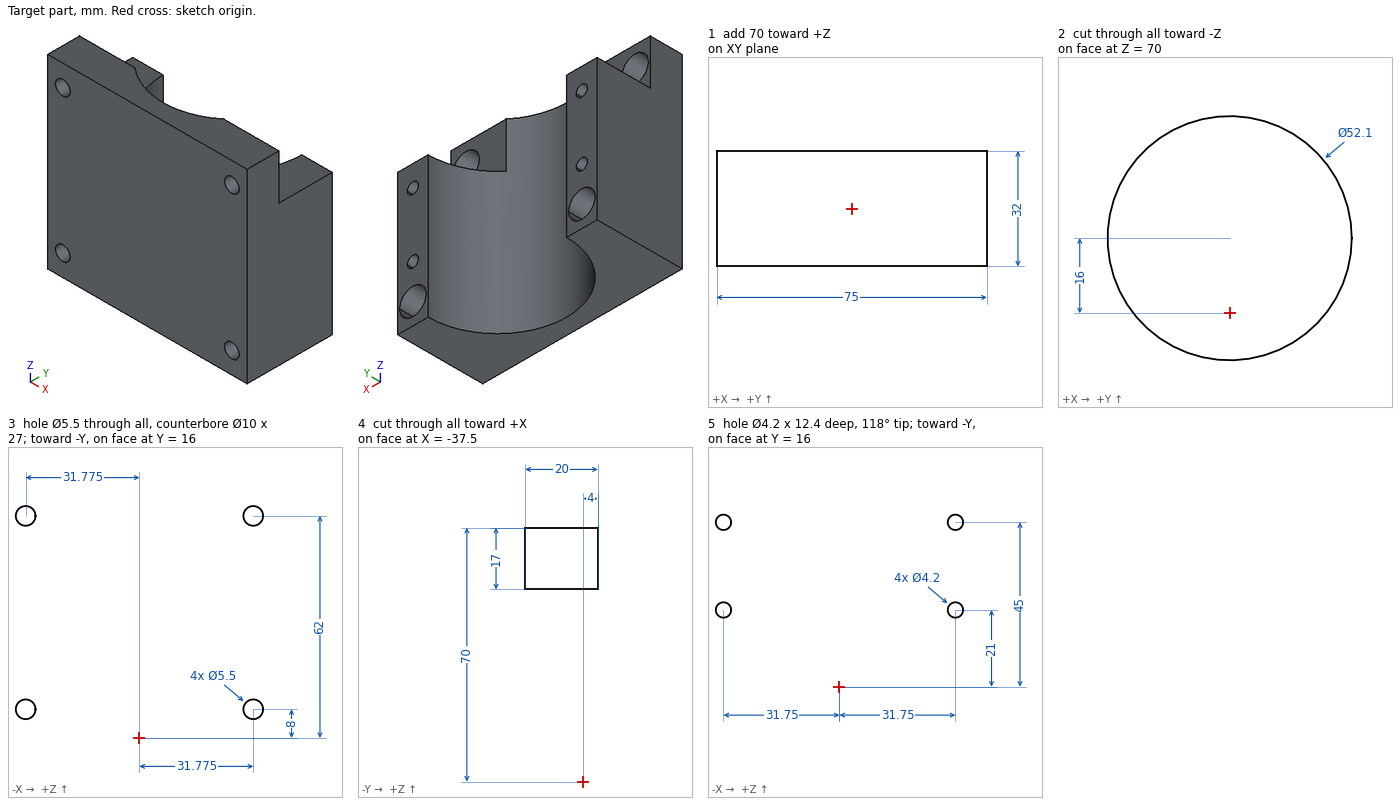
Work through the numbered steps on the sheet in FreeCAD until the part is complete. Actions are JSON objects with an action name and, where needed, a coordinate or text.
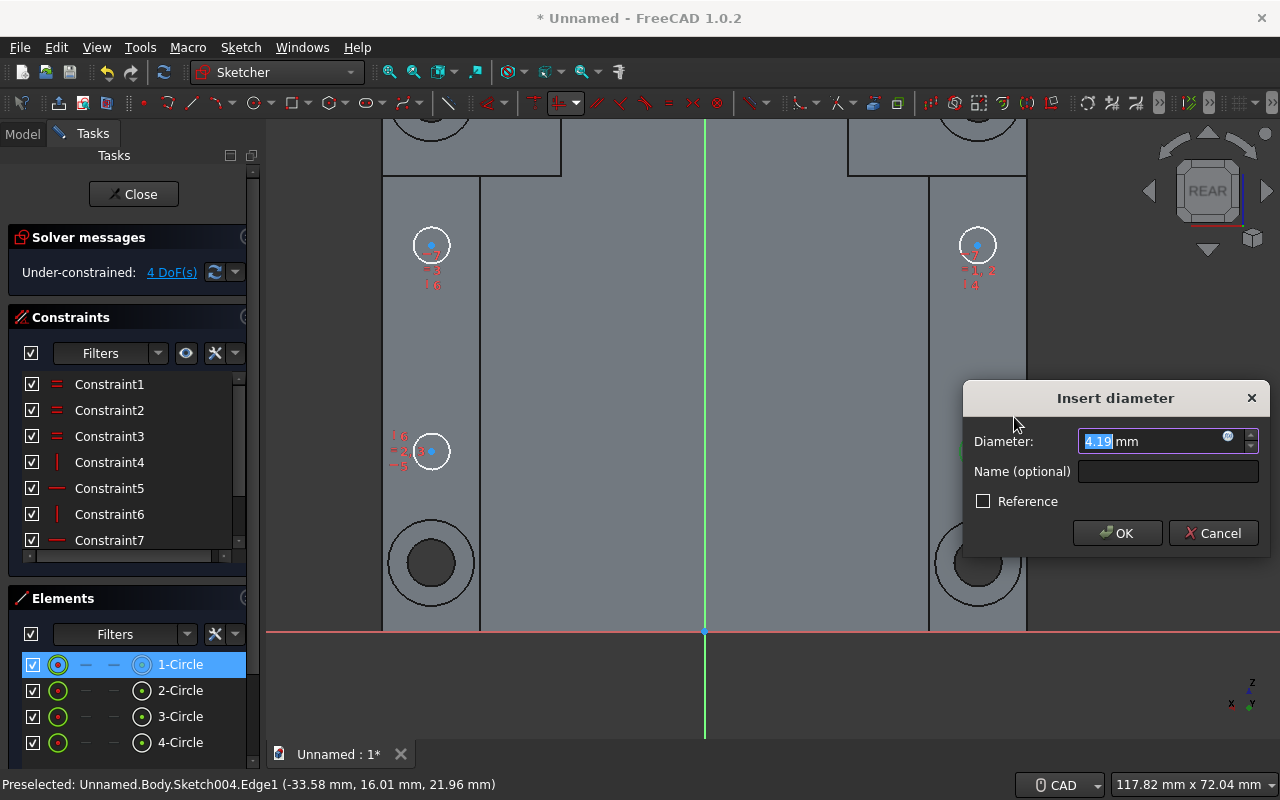
{"action": "type", "text": "4.2"}
{"action": "key", "text": "Return"}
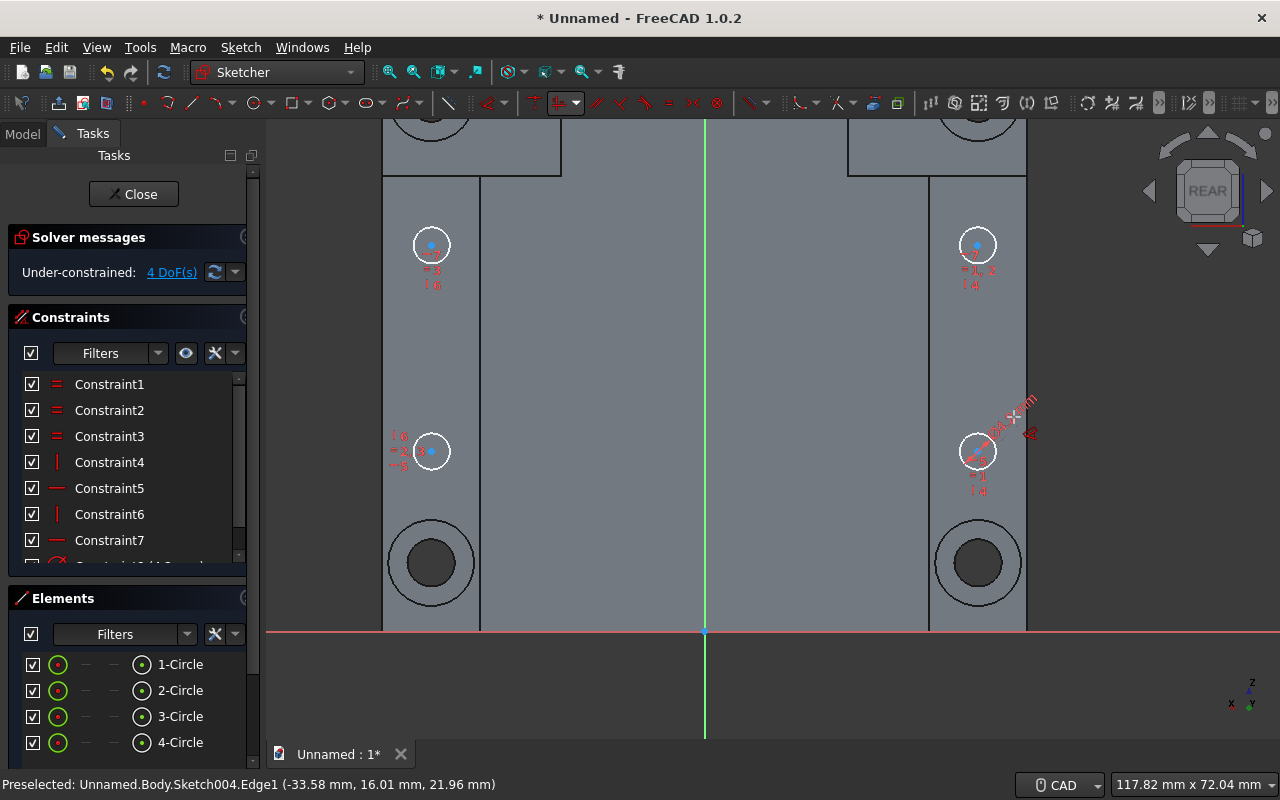
{"action": "left_click", "coordinate": [978, 452]}
{"action": "left_click", "coordinate": [1012, 542]}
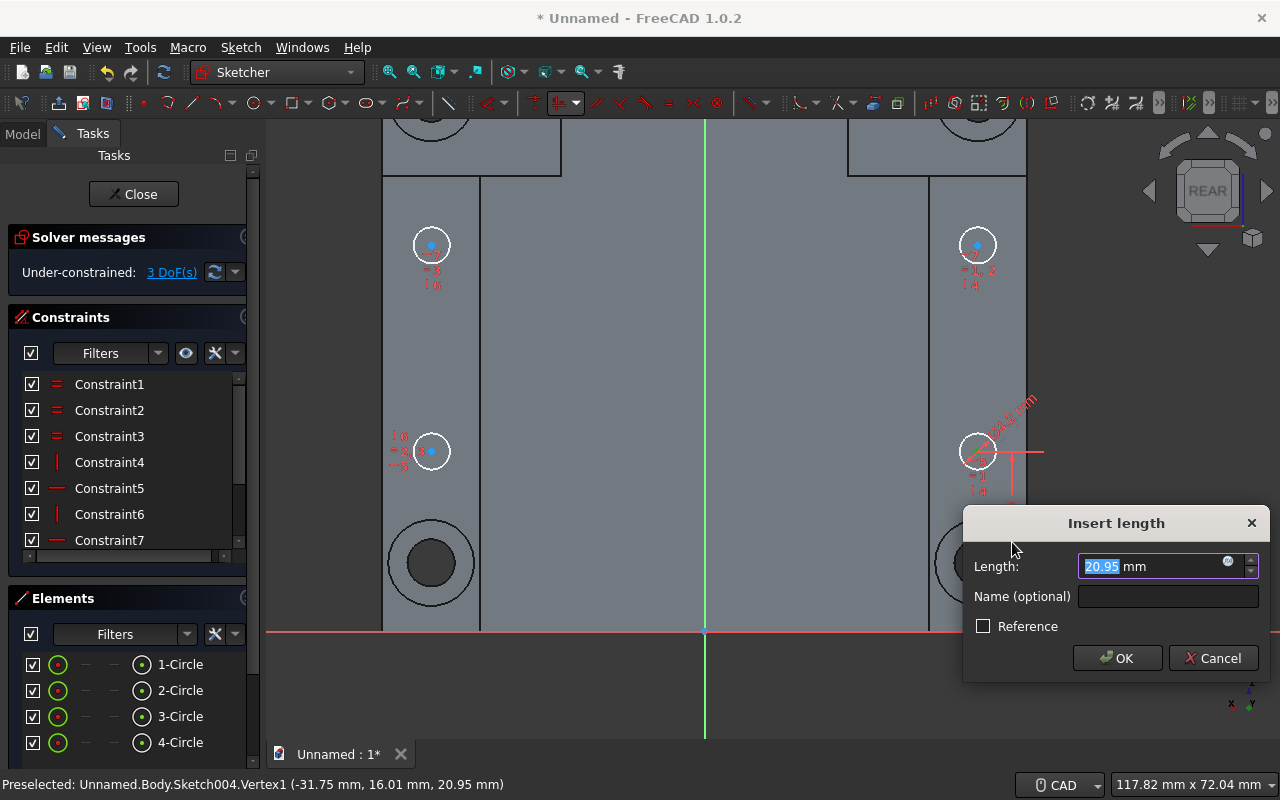
{"action": "type", "text": "21"}
{"action": "key", "text": "Return"}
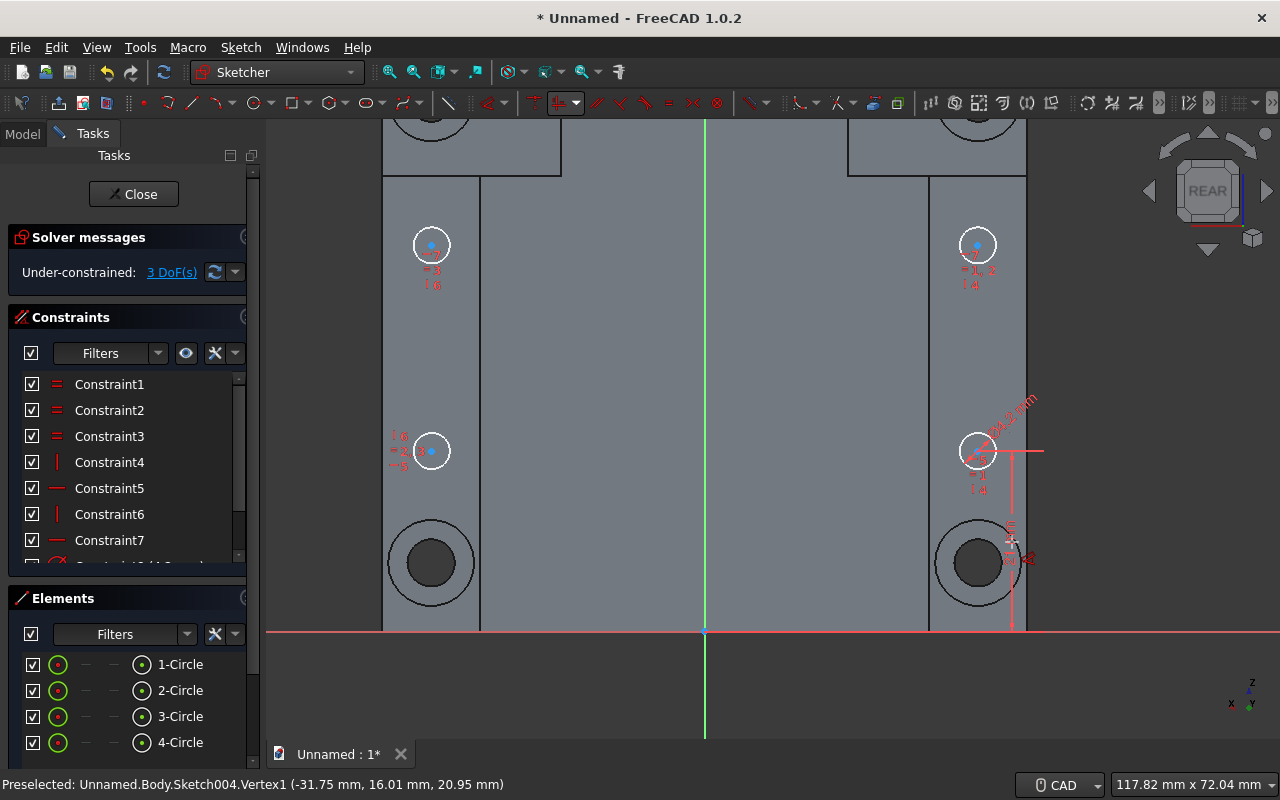
{"action": "left_click", "coordinate": [978, 245]}
{"action": "left_click", "coordinate": [1012, 439]}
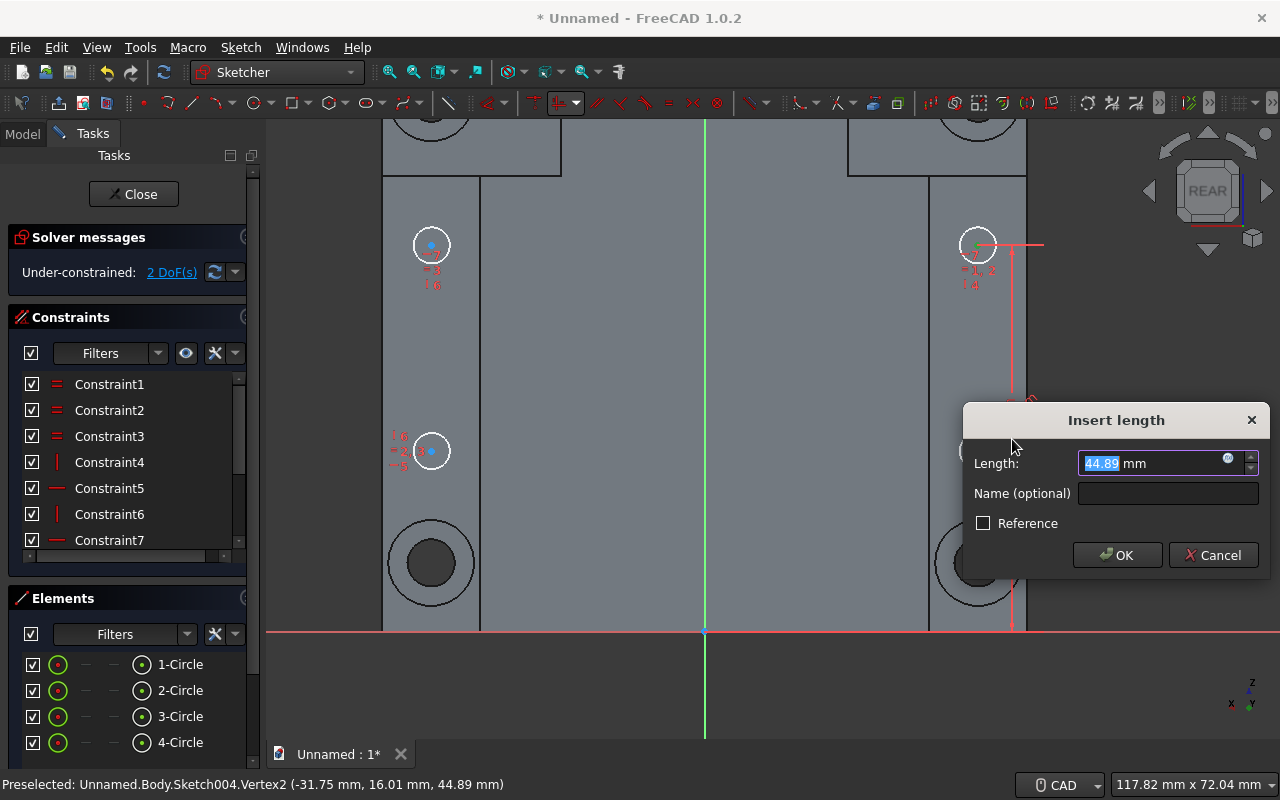
{"action": "type", "text": "45"}
{"action": "key", "text": "Return"}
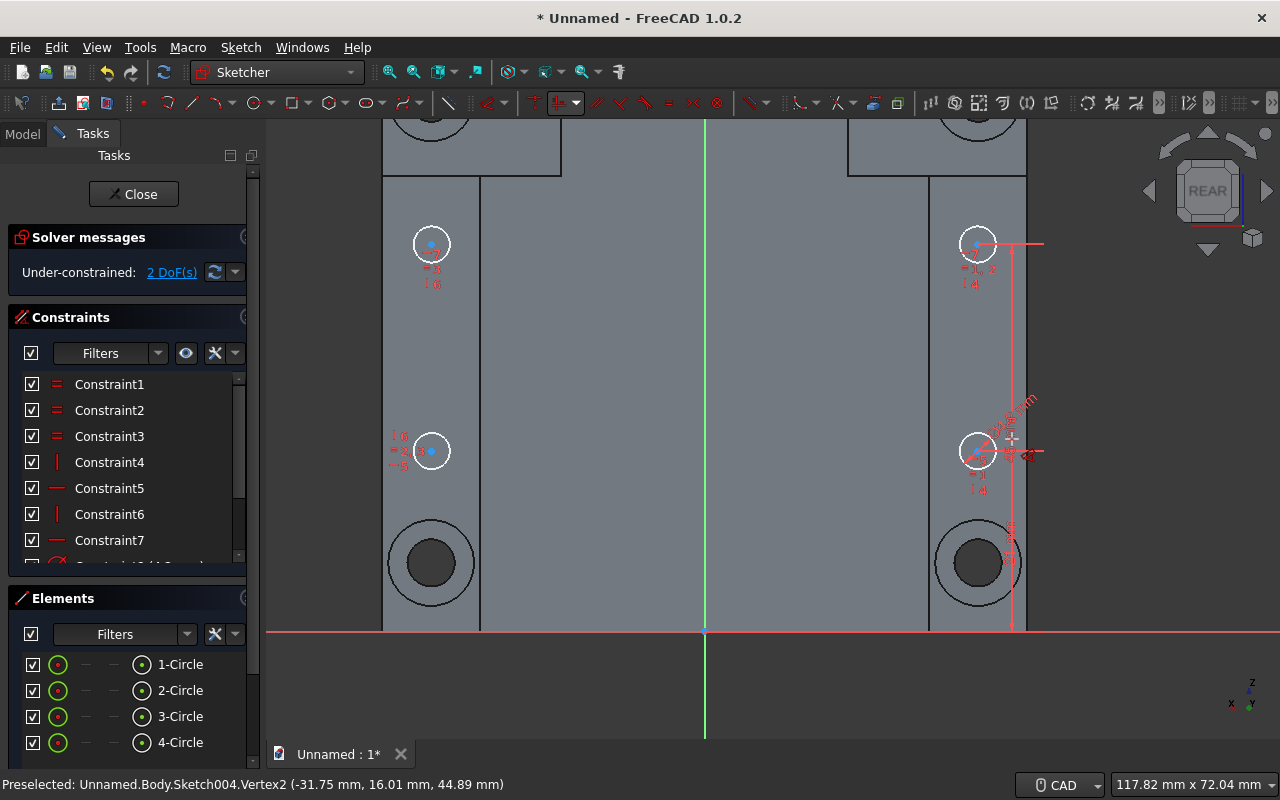
{"action": "left_click", "coordinate": [978, 451]}
{"action": "left_click", "coordinate": [841, 666]}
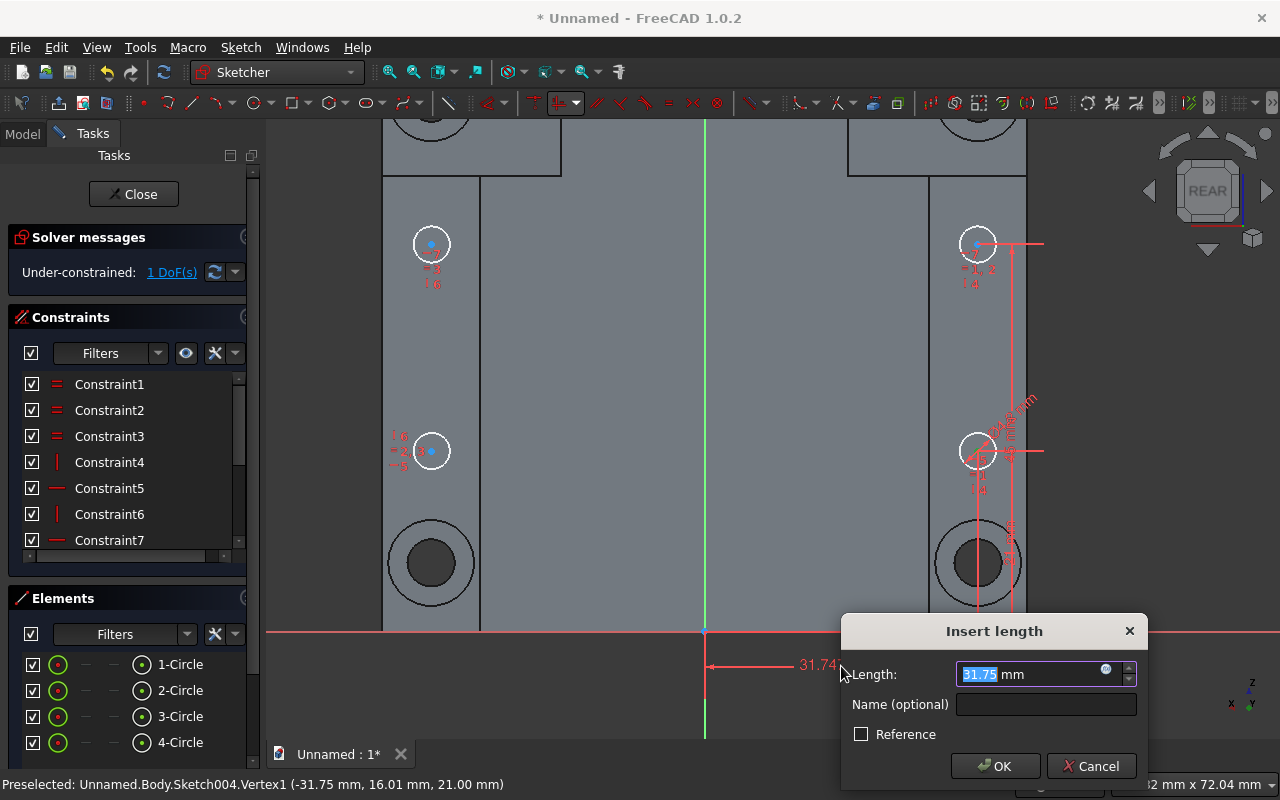
{"action": "type", "text": "31.75"}
{"action": "key", "text": "Return"}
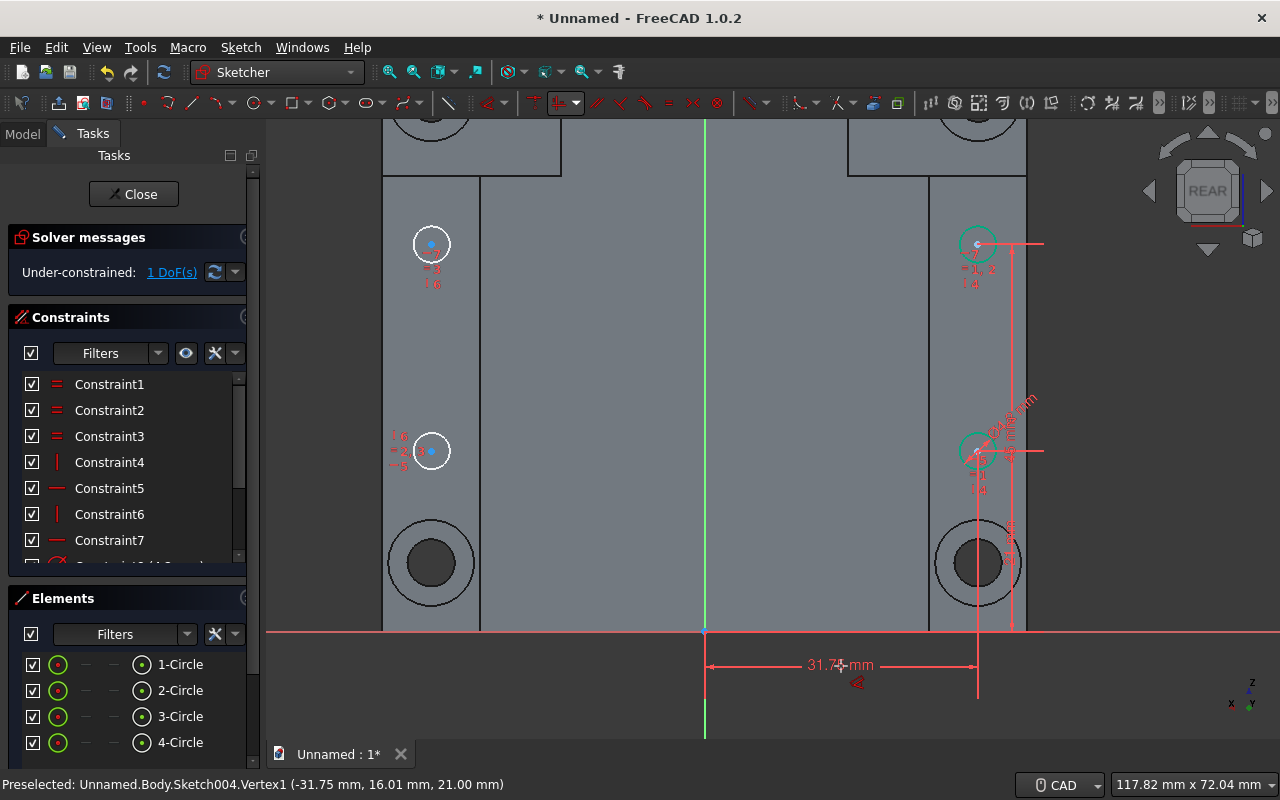
{"action": "left_click", "coordinate": [432, 451]}
{"action": "left_click", "coordinate": [568, 666]}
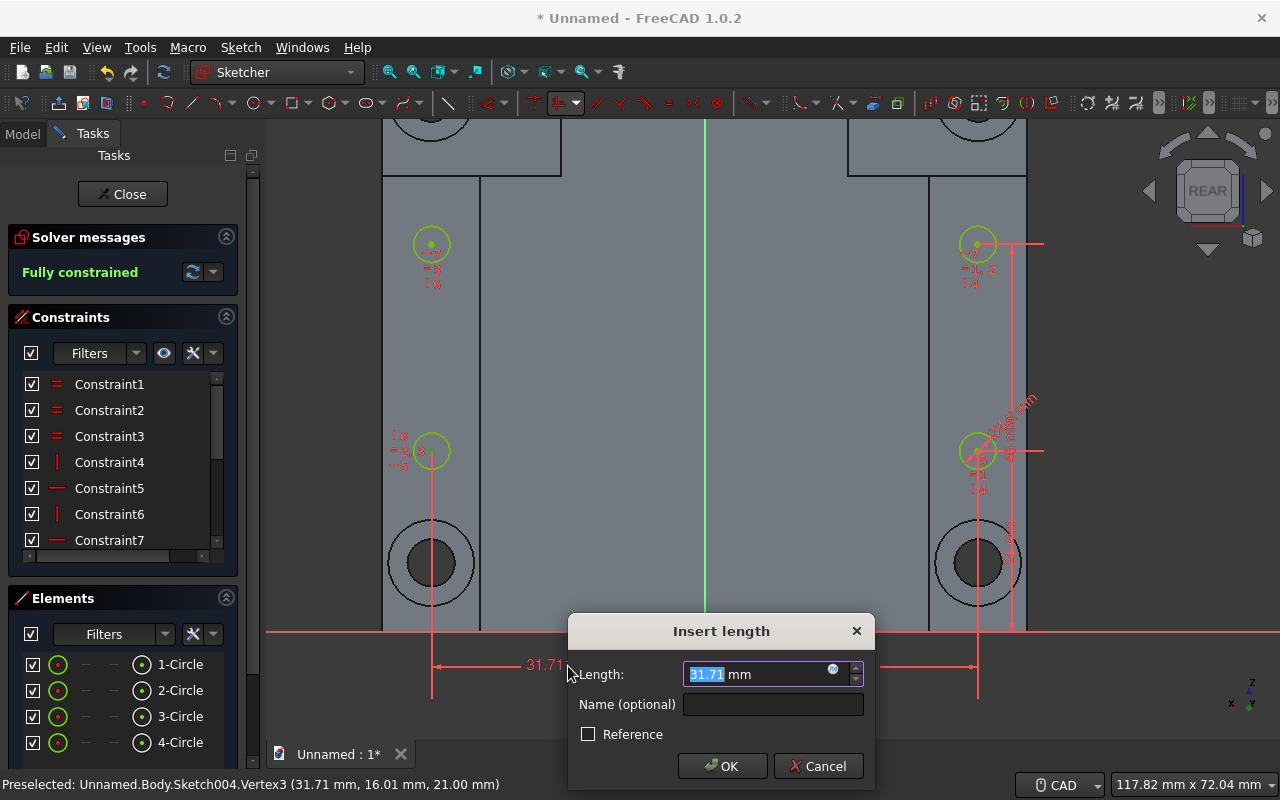
{"action": "type", "text": "31.75"}
{"action": "key", "text": "Return"}
{"action": "key", "text": "Escape"}